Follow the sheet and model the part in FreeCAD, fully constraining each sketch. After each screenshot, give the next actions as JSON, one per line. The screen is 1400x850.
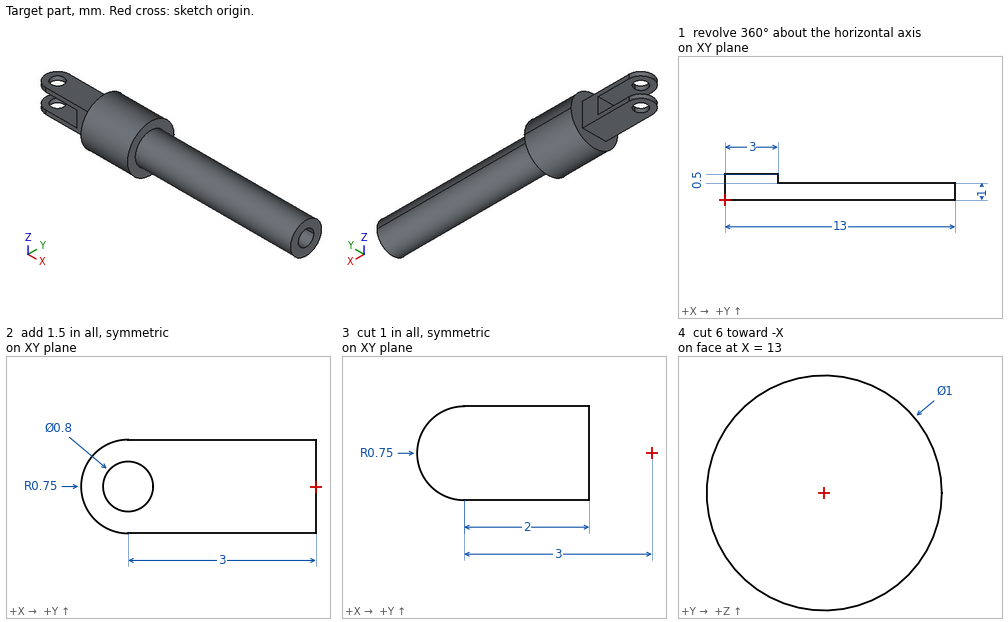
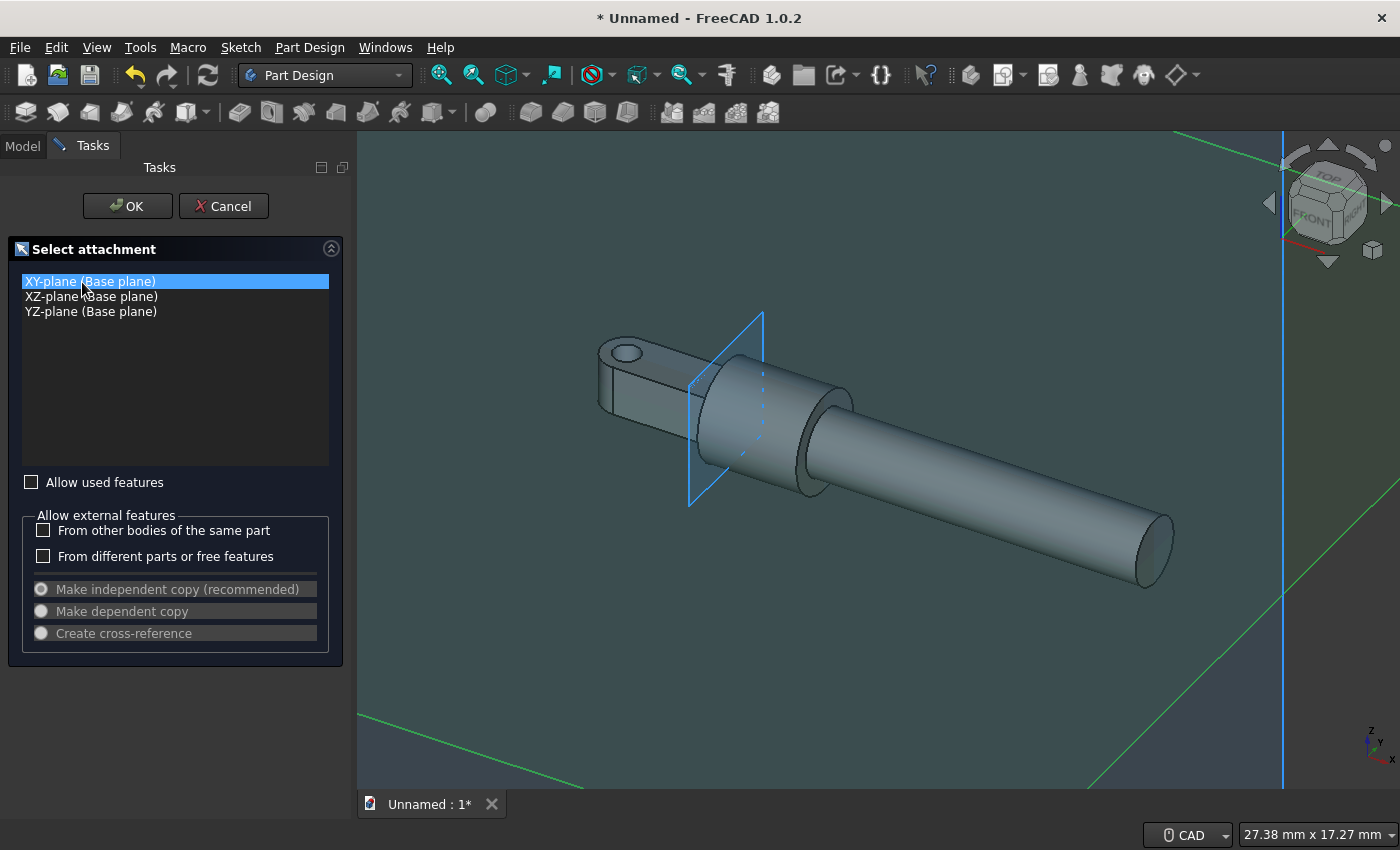
{"action": "left_click", "coordinate": [128, 206]}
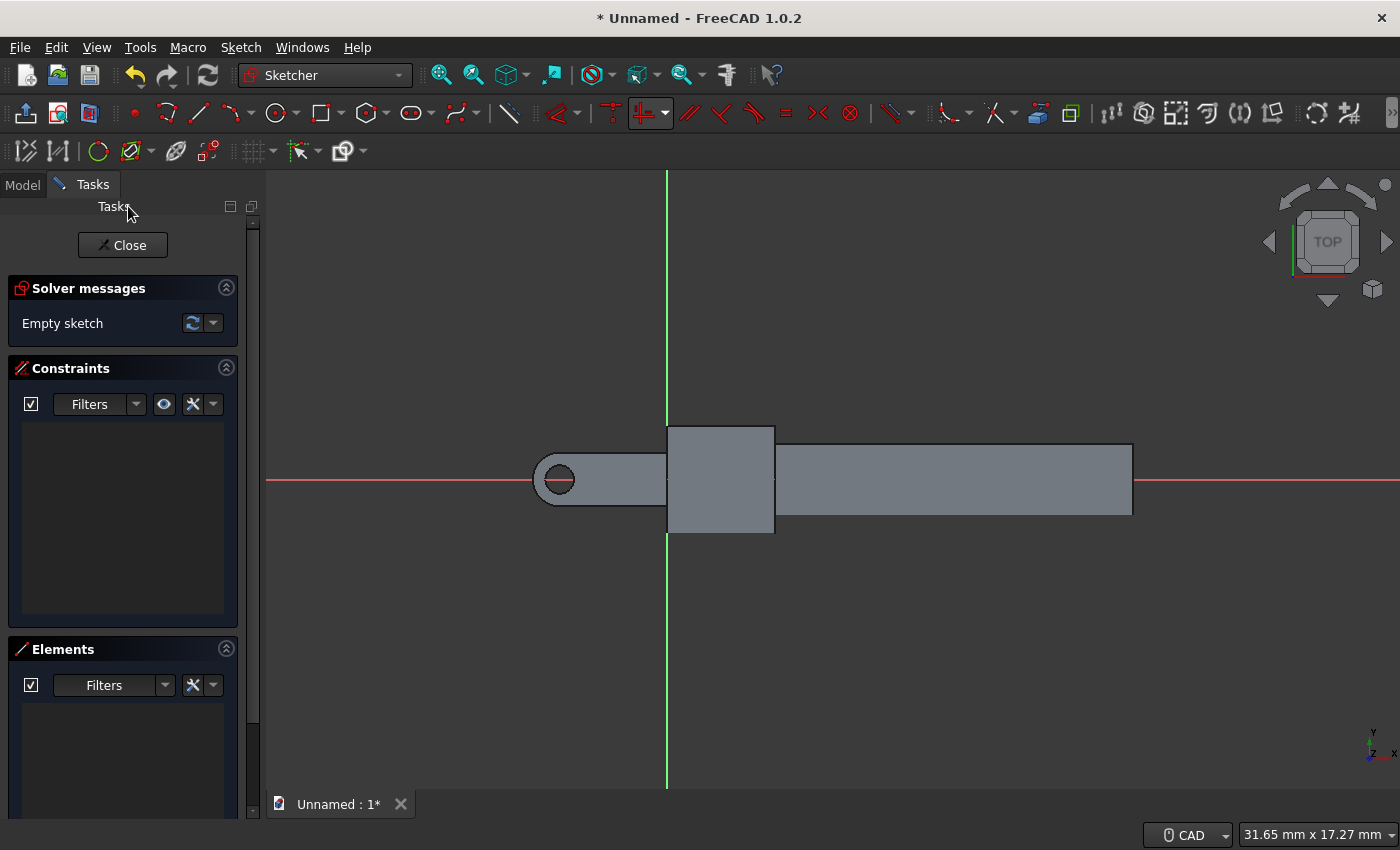
{"action": "left_click", "coordinate": [90, 114]}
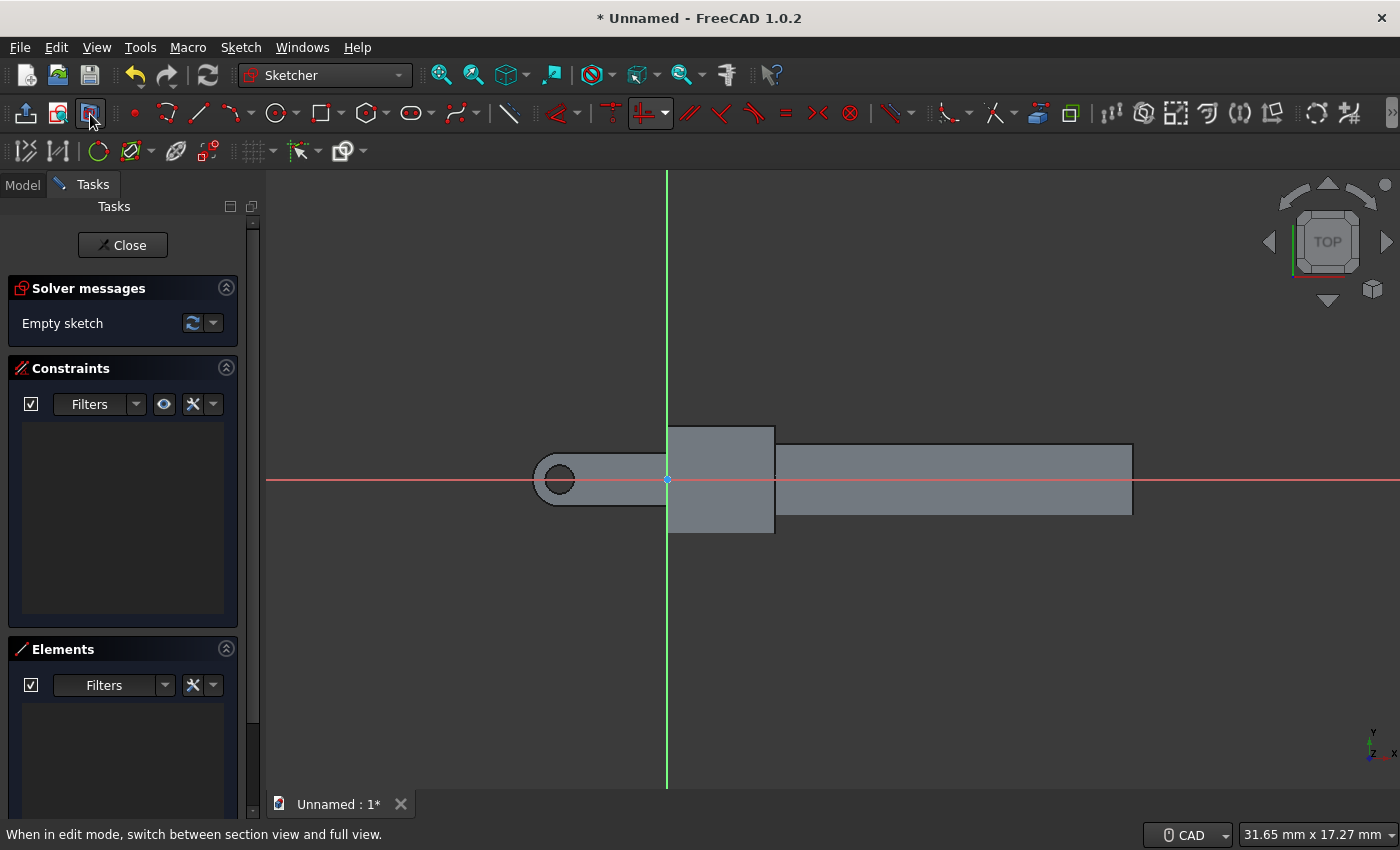
{"action": "scroll", "coordinate": [558, 479], "scroll_direction": "up", "scroll_amount": 8}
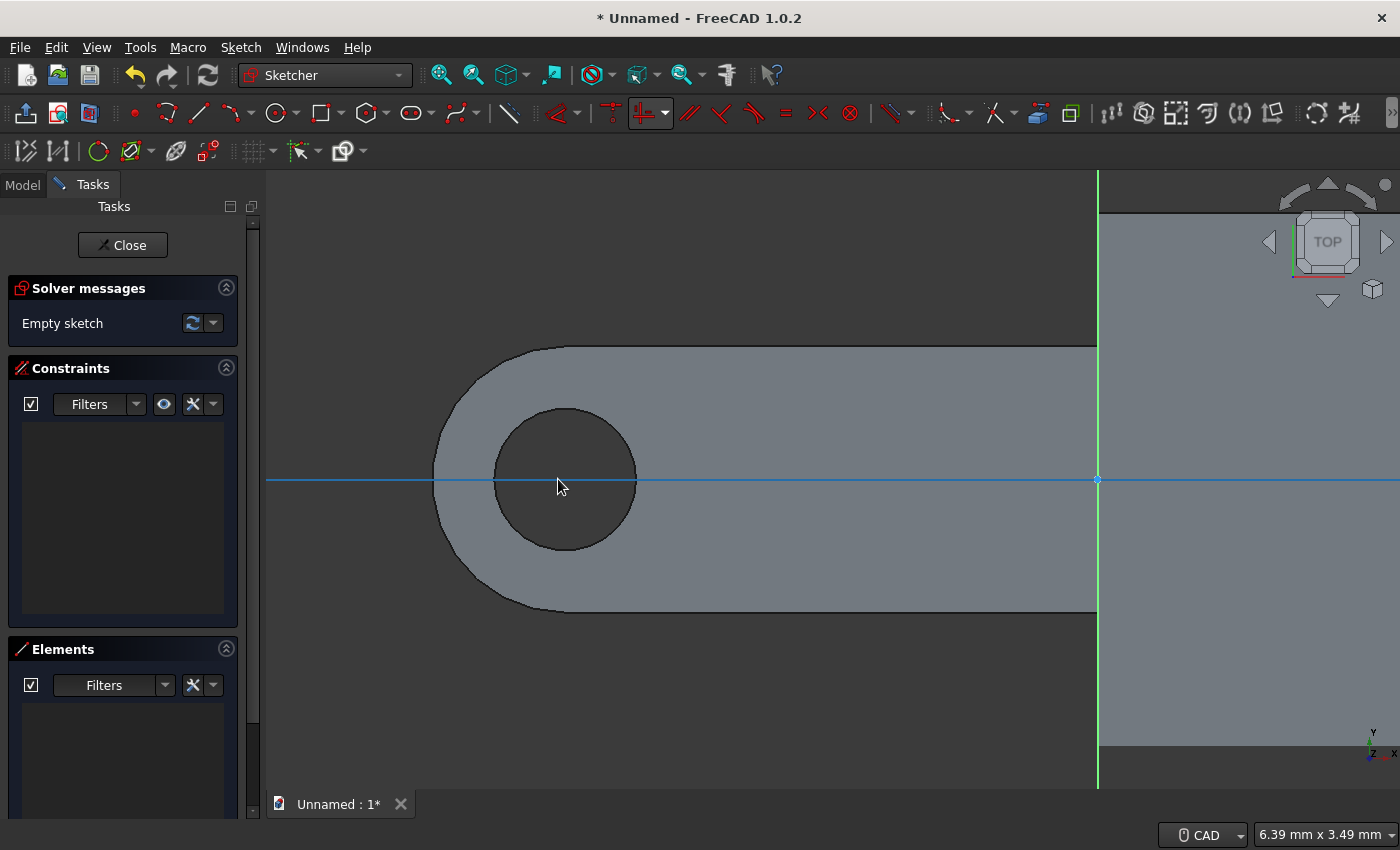
{"action": "left_click", "coordinate": [168, 114]}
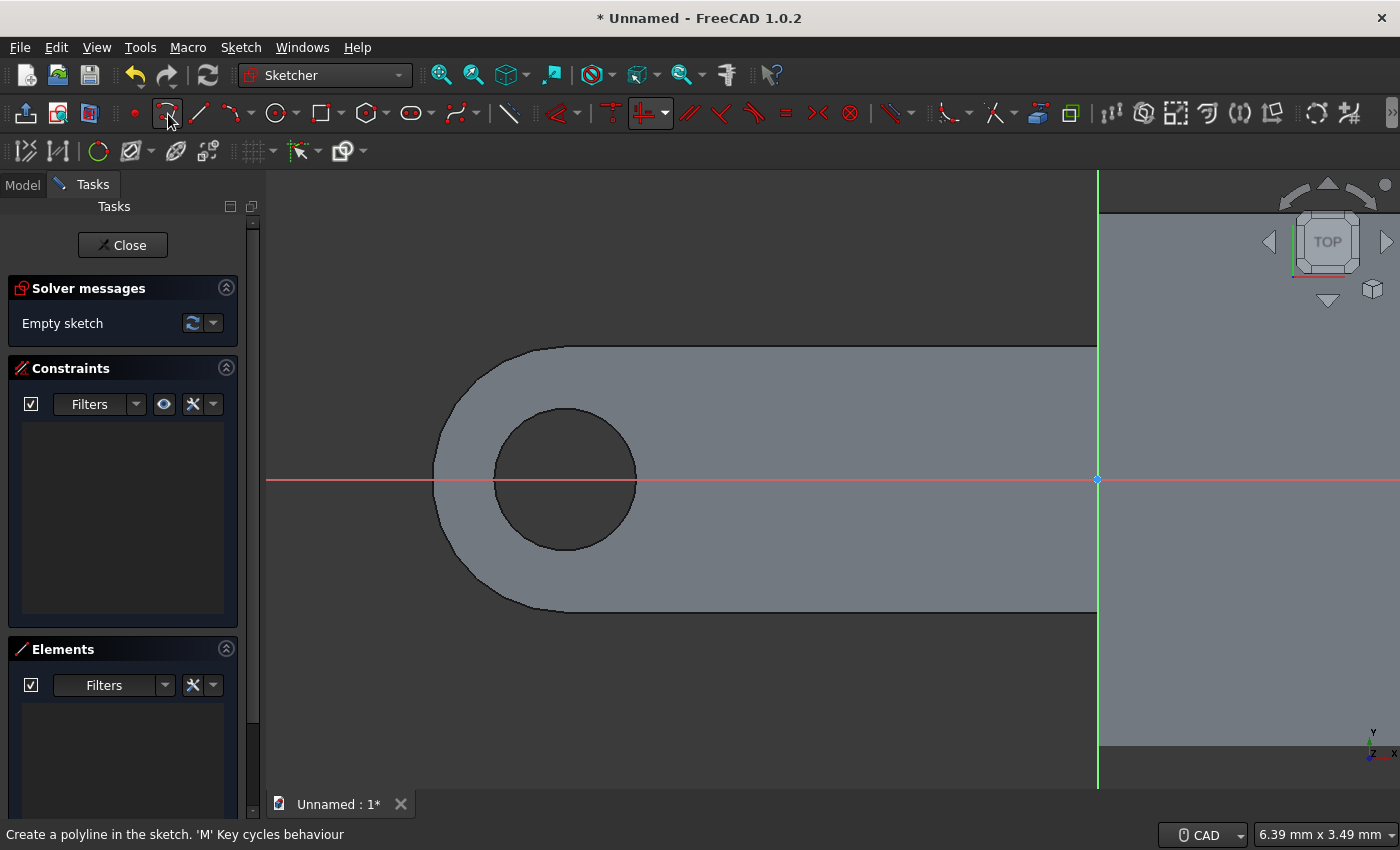
{"action": "left_click", "coordinate": [565, 613]}
{"action": "left_click", "coordinate": [920, 613]}
{"action": "left_click", "coordinate": [920, 346]}
{"action": "left_click", "coordinate": [565, 346]}
{"action": "right_click", "coordinate": [565, 346]}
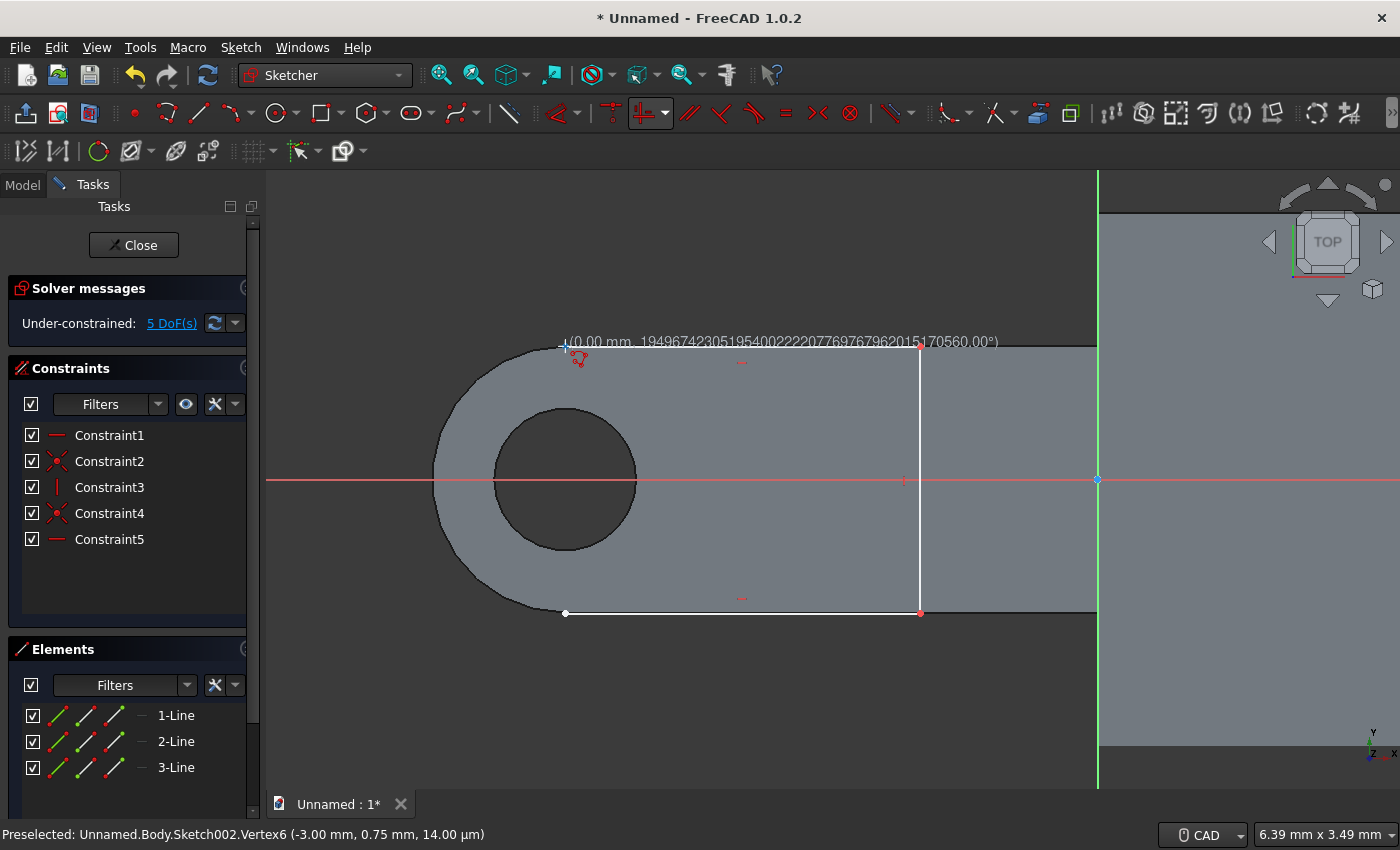
{"action": "left_click", "coordinate": [232, 114]}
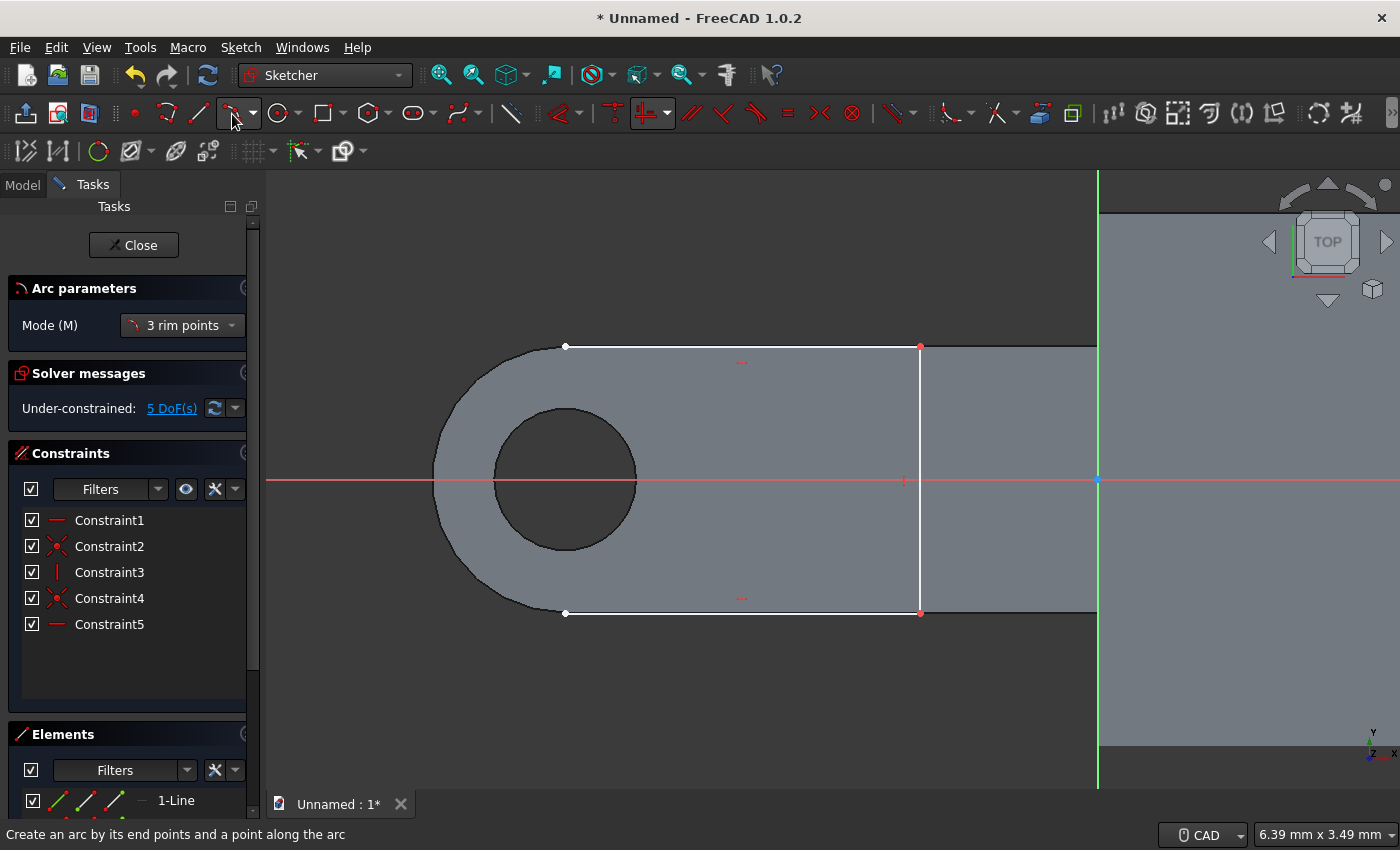
{"action": "left_click", "coordinate": [565, 347]}
{"action": "left_click", "coordinate": [565, 614]}
{"action": "left_click", "coordinate": [439, 438]}
{"action": "key", "text": "Escape"}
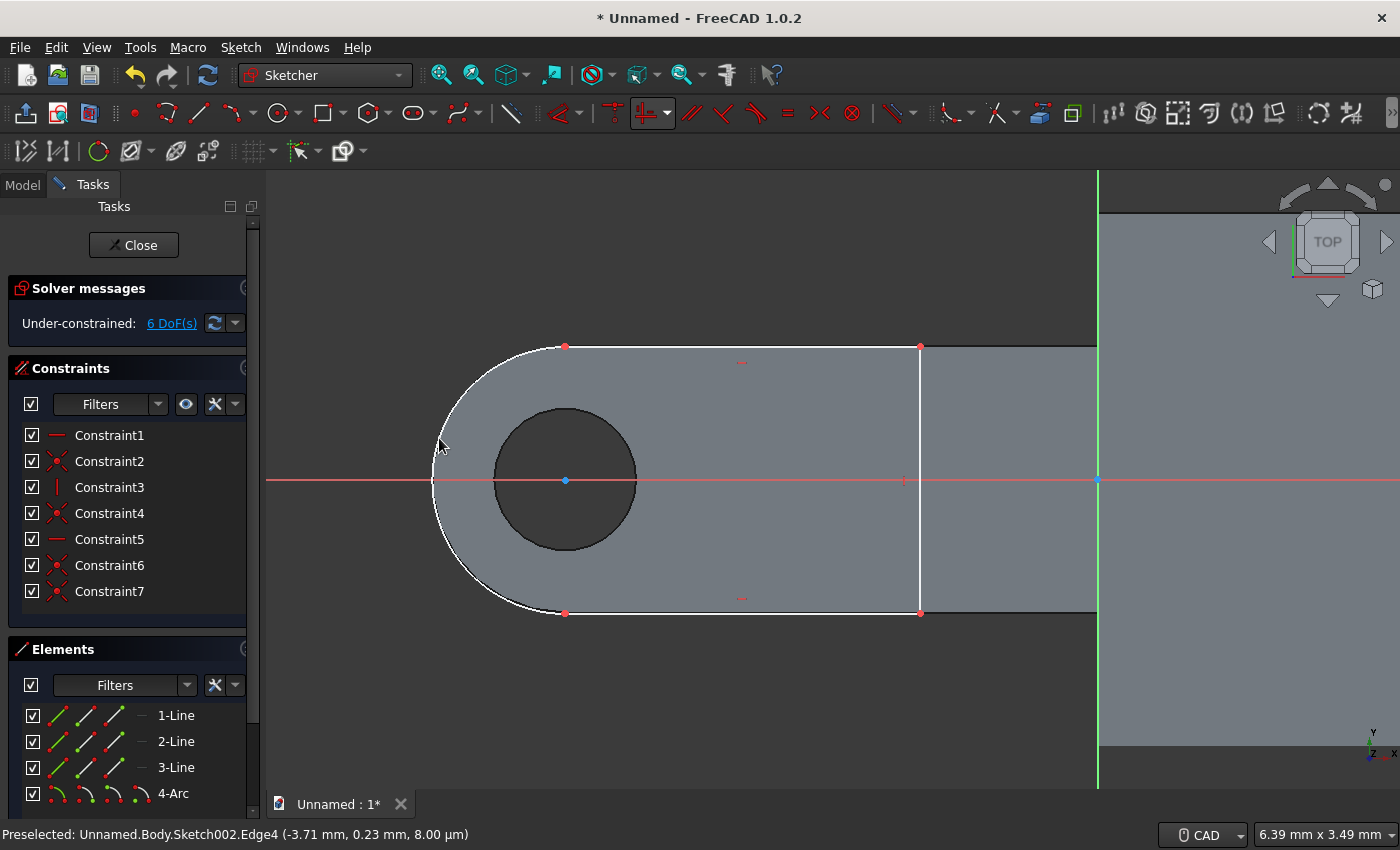
{"action": "left_click", "coordinate": [671, 614]}